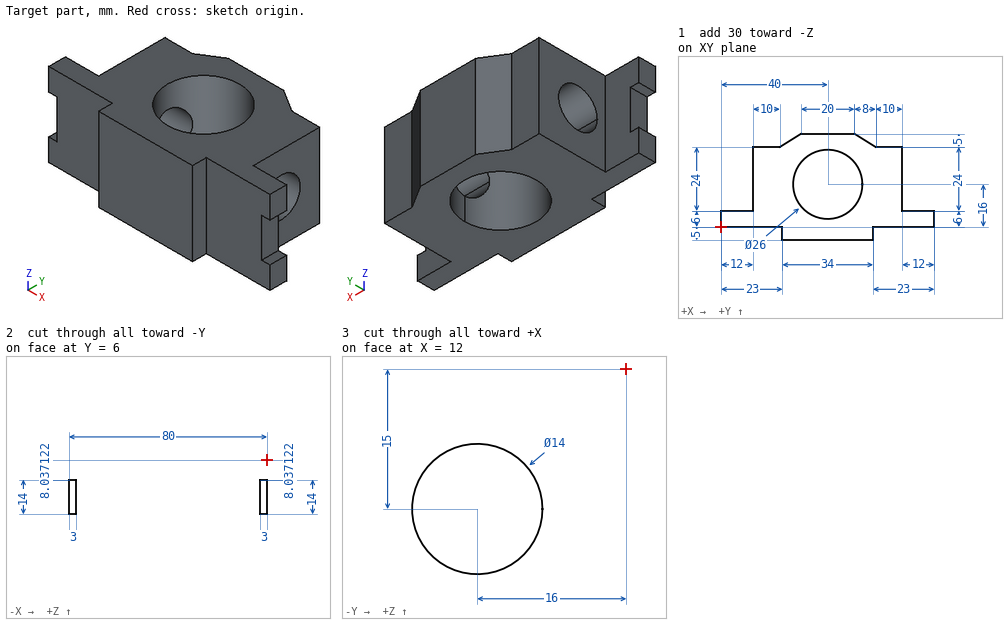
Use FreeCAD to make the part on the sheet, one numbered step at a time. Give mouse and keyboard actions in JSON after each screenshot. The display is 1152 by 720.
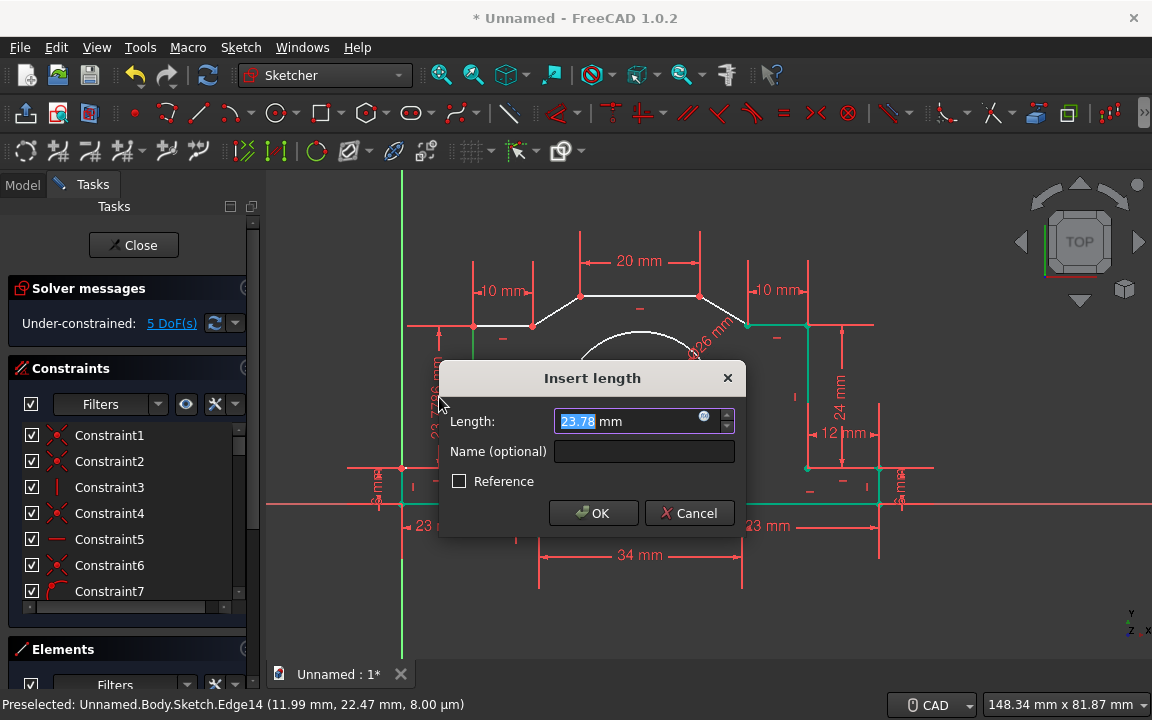
{"action": "type", "text": "24"}
{"action": "key", "text": "Return"}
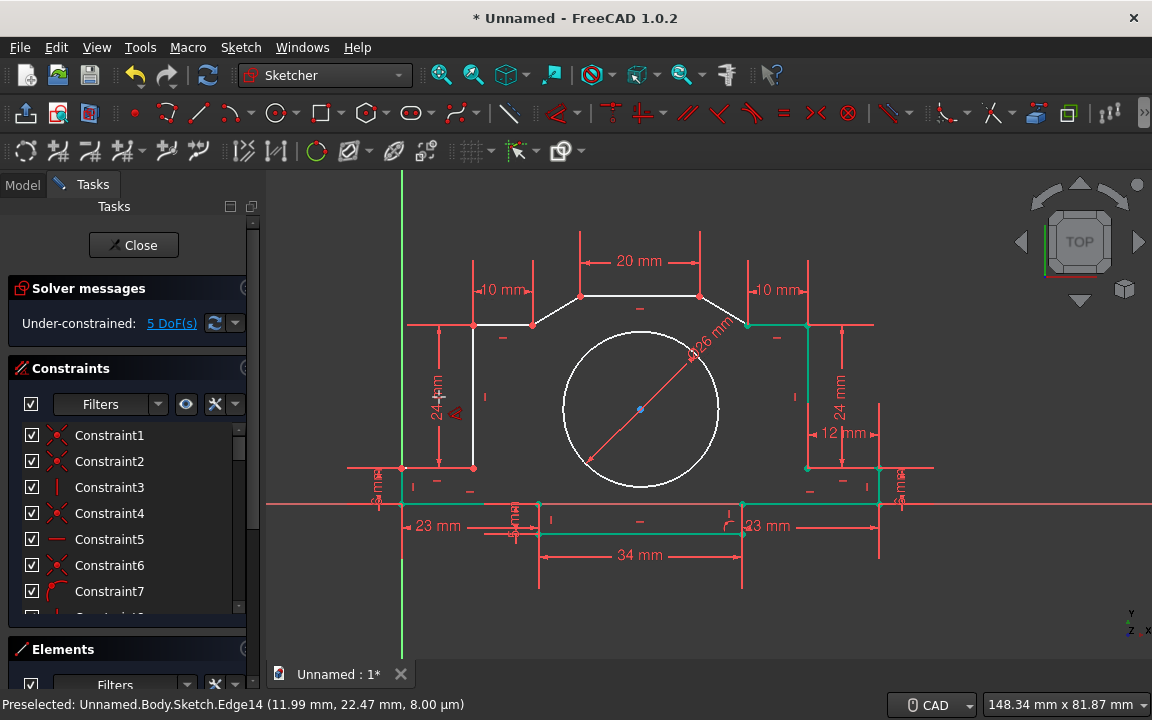
{"action": "left_click", "coordinate": [452, 468]}
{"action": "left_click", "coordinate": [437, 434]}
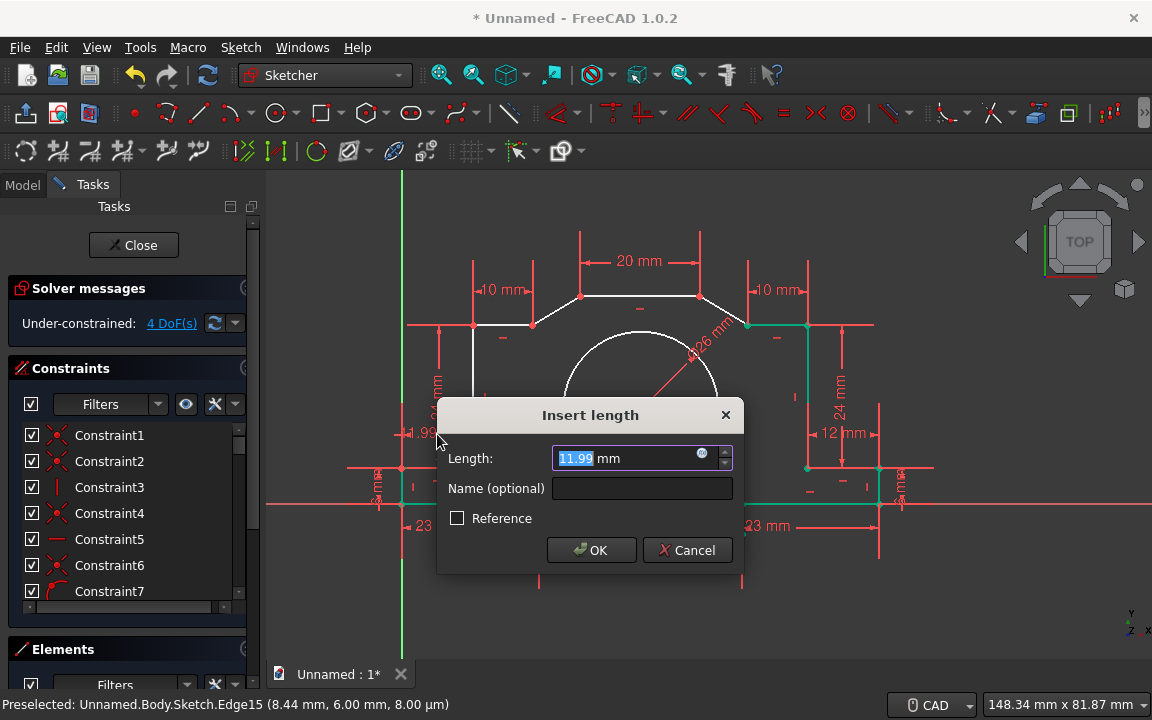
{"action": "type", "text": "12"}
{"action": "key", "text": "Return"}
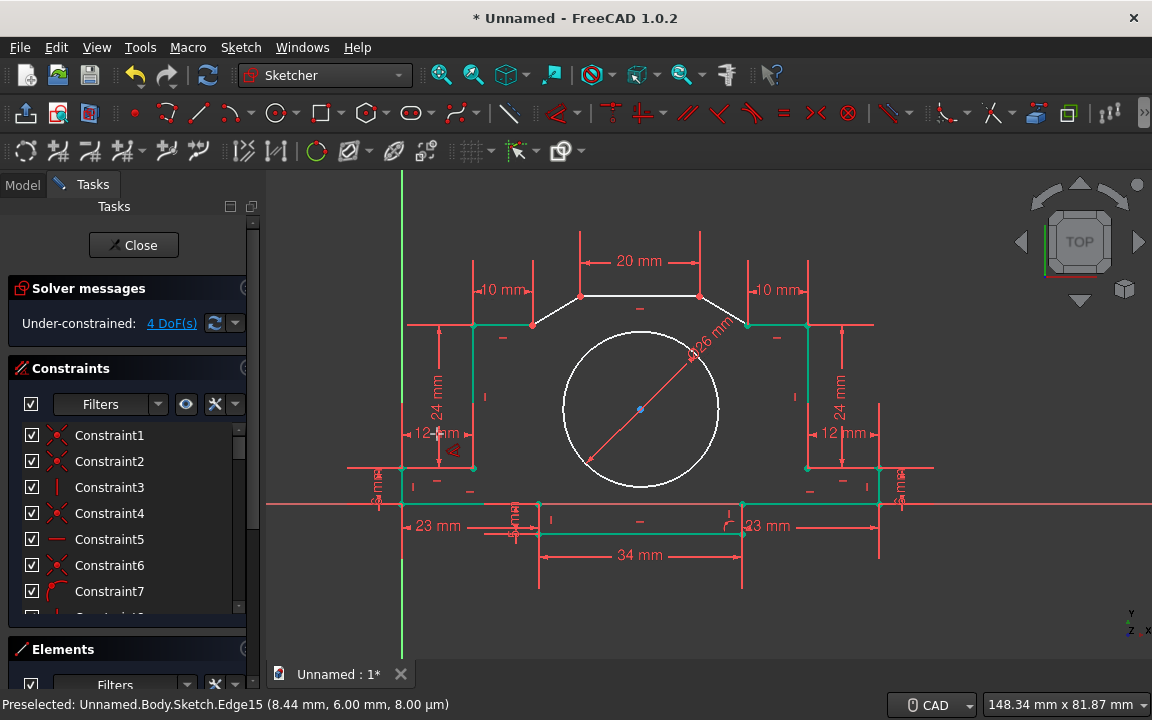
{"action": "left_click", "coordinate": [734, 316]}
{"action": "left_click", "coordinate": [724, 262]}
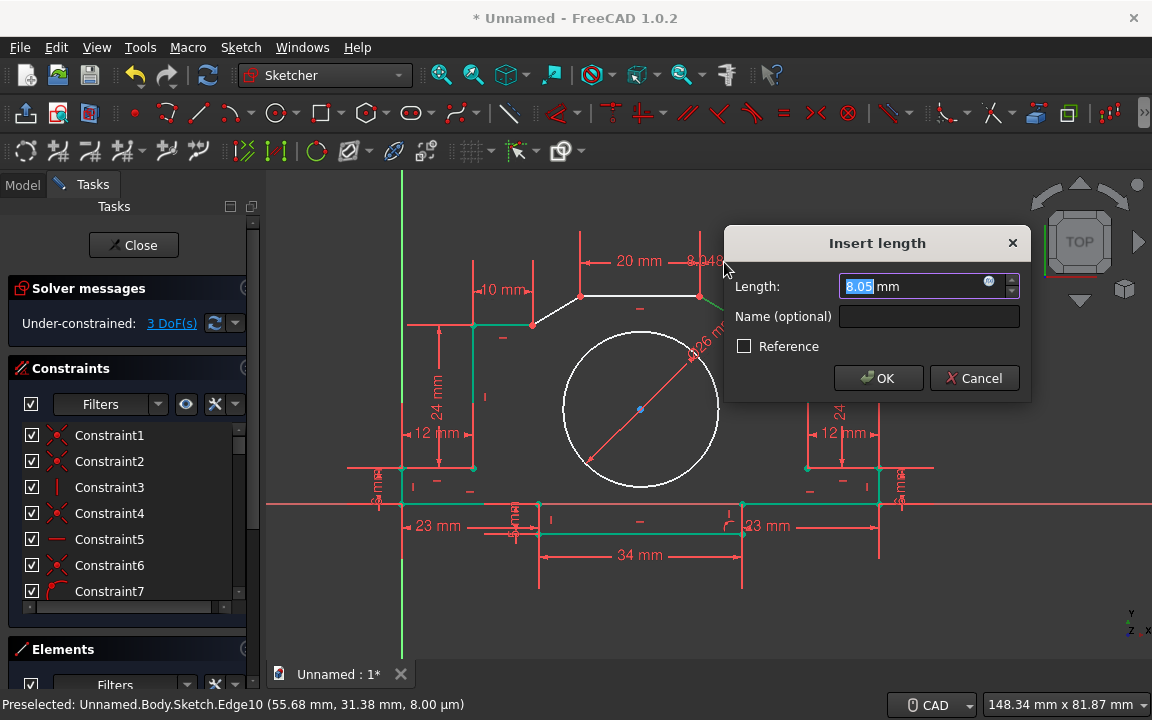
{"action": "type", "text": "8"}
{"action": "key", "text": "Return"}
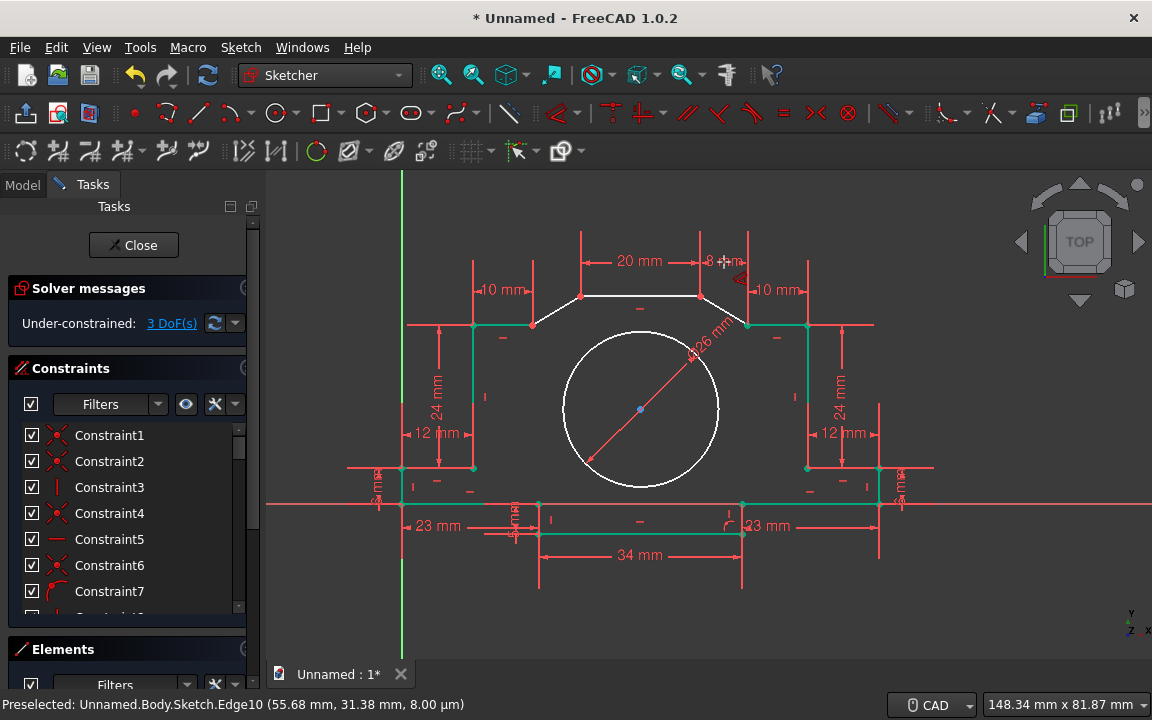
{"action": "scroll", "coordinate": [734, 316], "scroll_direction": "up", "scroll_amount": 2}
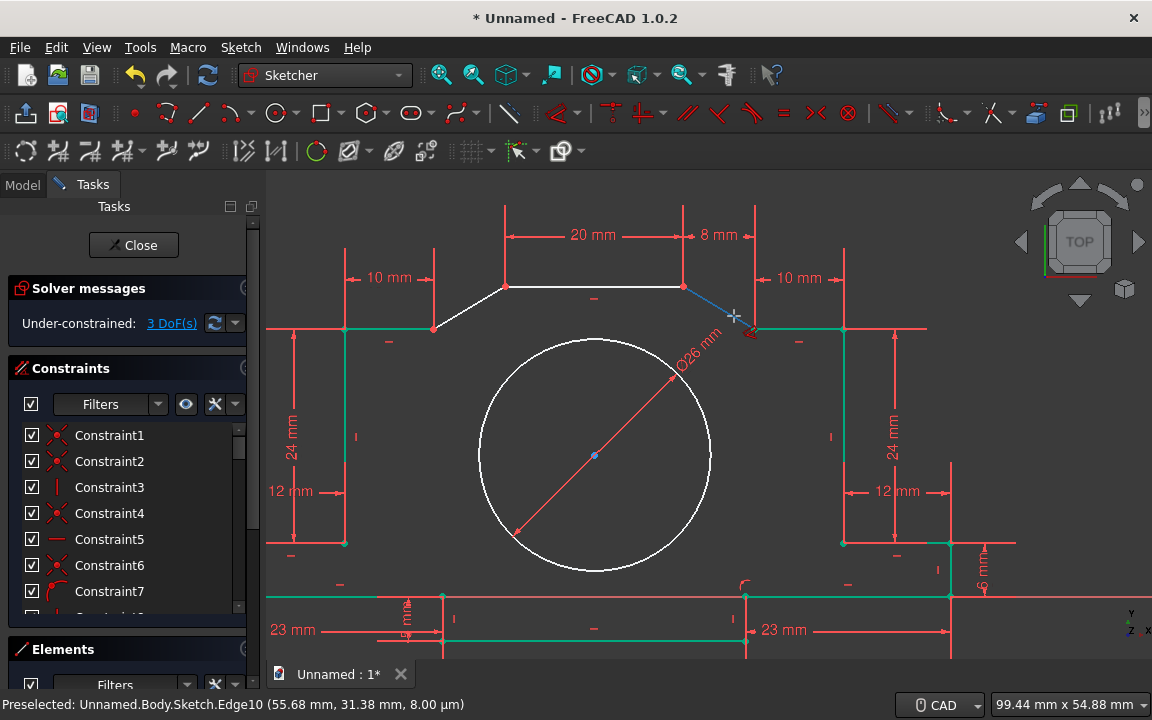
{"action": "left_click", "coordinate": [733, 316]}
{"action": "left_click", "coordinate": [789, 308]}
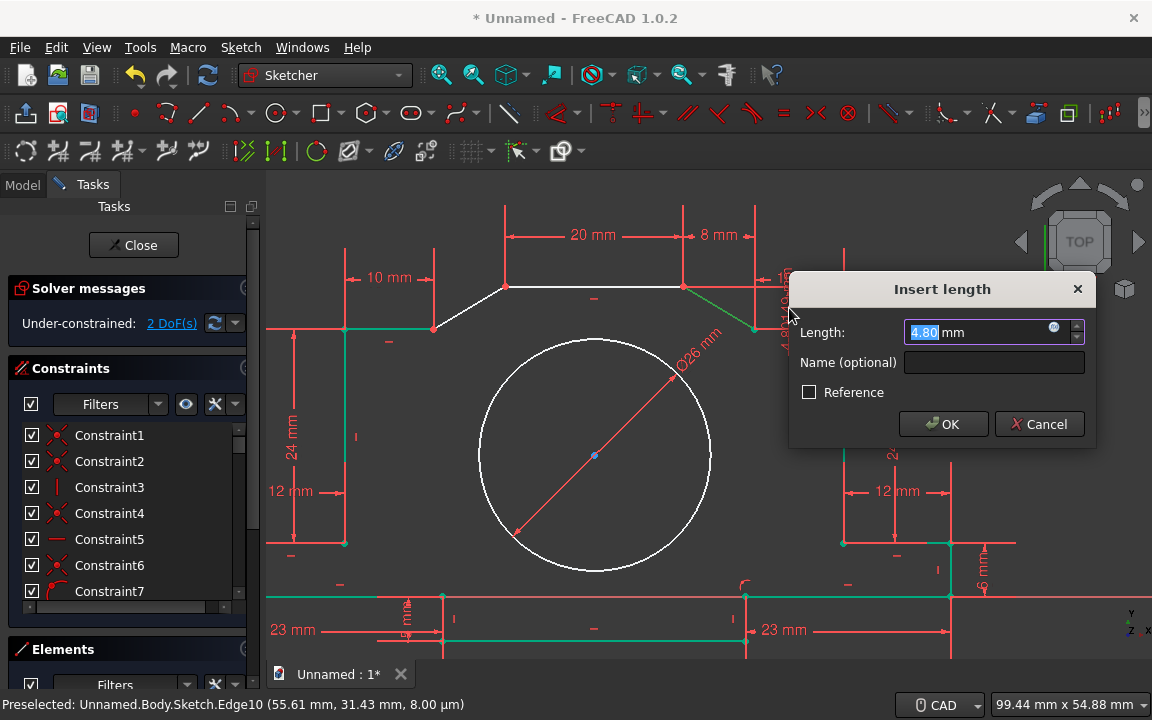
{"action": "type", "text": "5"}
{"action": "key", "text": "Return"}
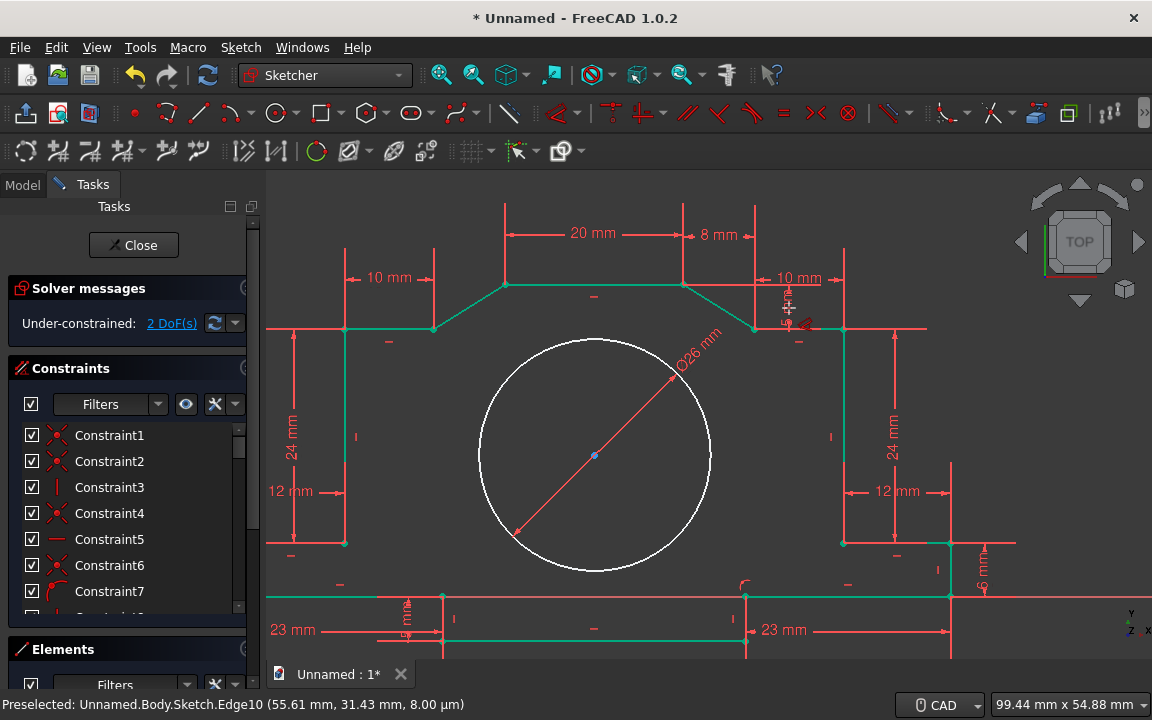
{"action": "left_click", "coordinate": [595, 455]}
{"action": "left_click", "coordinate": [444, 421]}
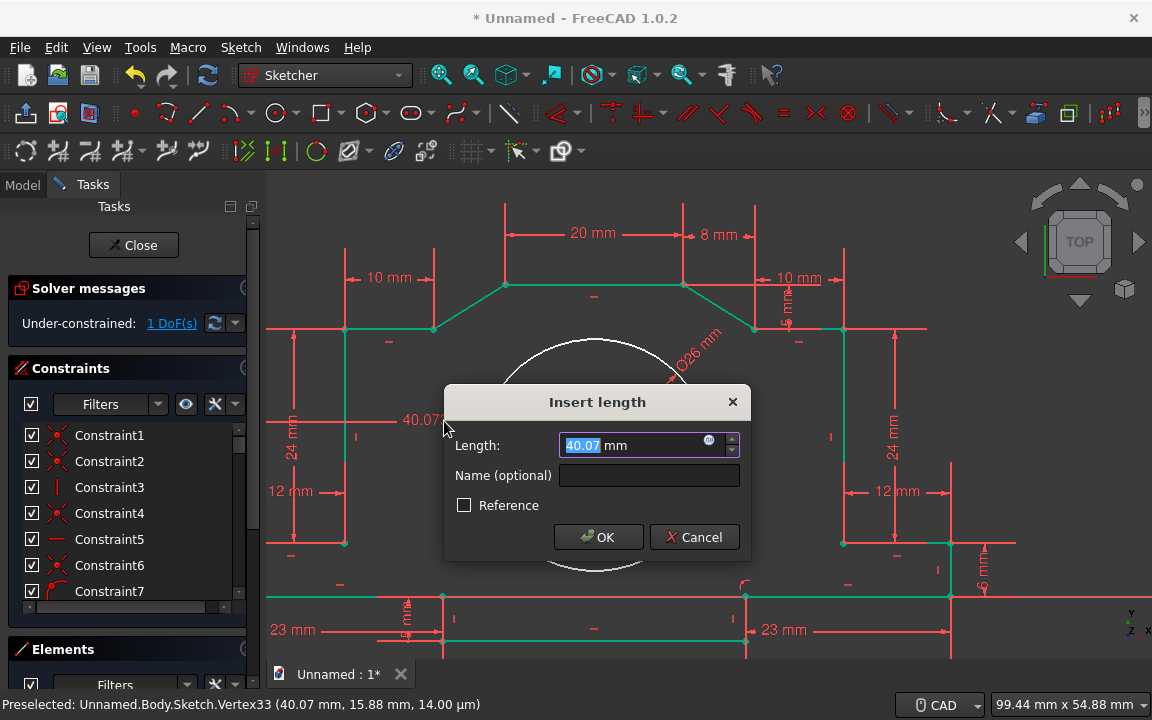
{"action": "type", "text": "40"}
{"action": "key", "text": "Return"}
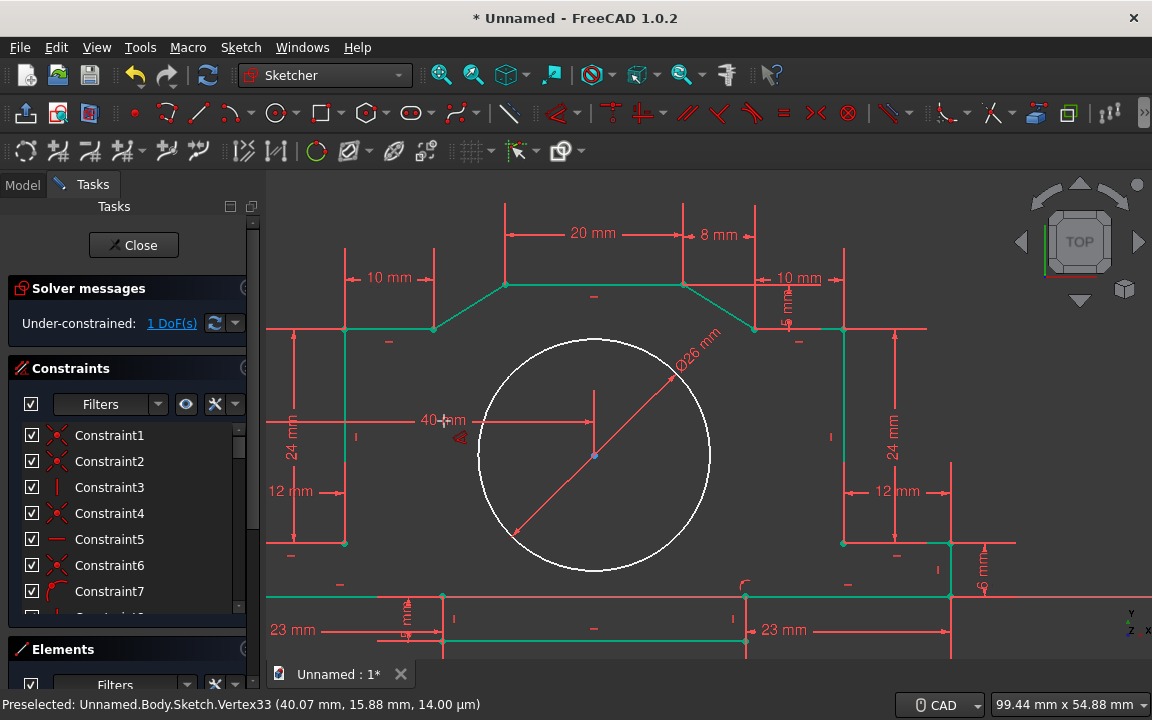
{"action": "left_click", "coordinate": [594, 455]}
{"action": "left_click", "coordinate": [628, 526]}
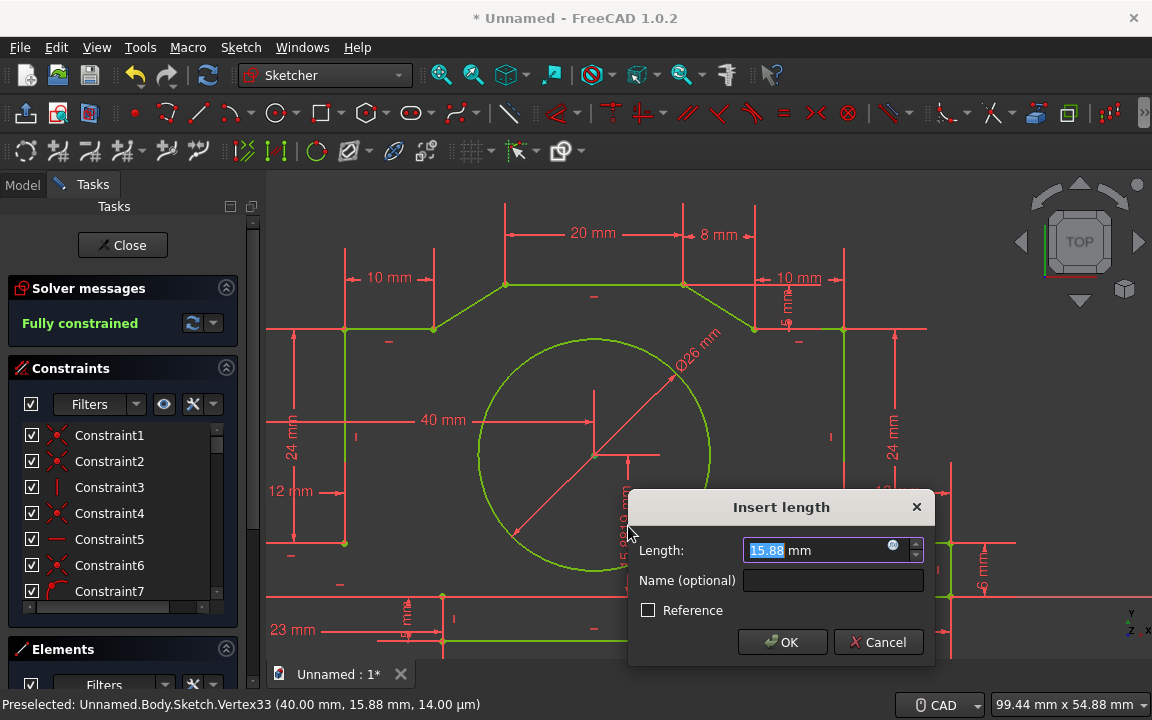
{"action": "type", "text": "16"}
{"action": "key", "text": "Return"}
{"action": "key", "text": "Escape"}